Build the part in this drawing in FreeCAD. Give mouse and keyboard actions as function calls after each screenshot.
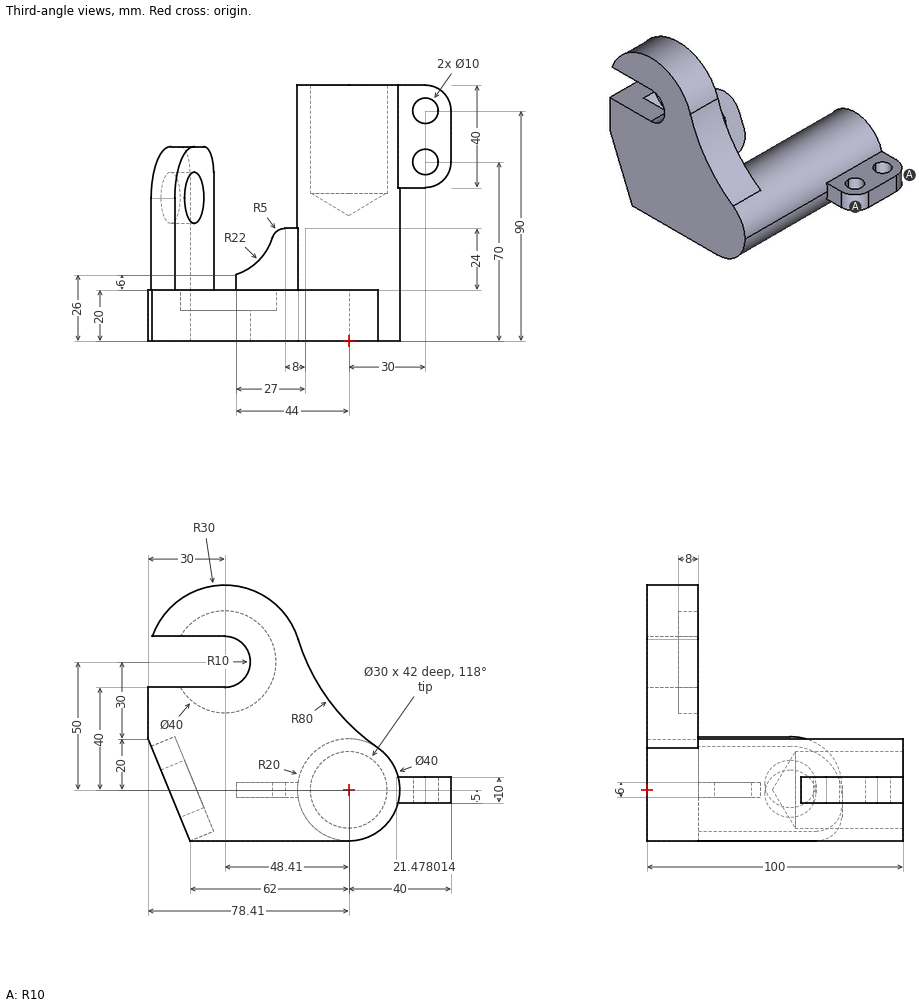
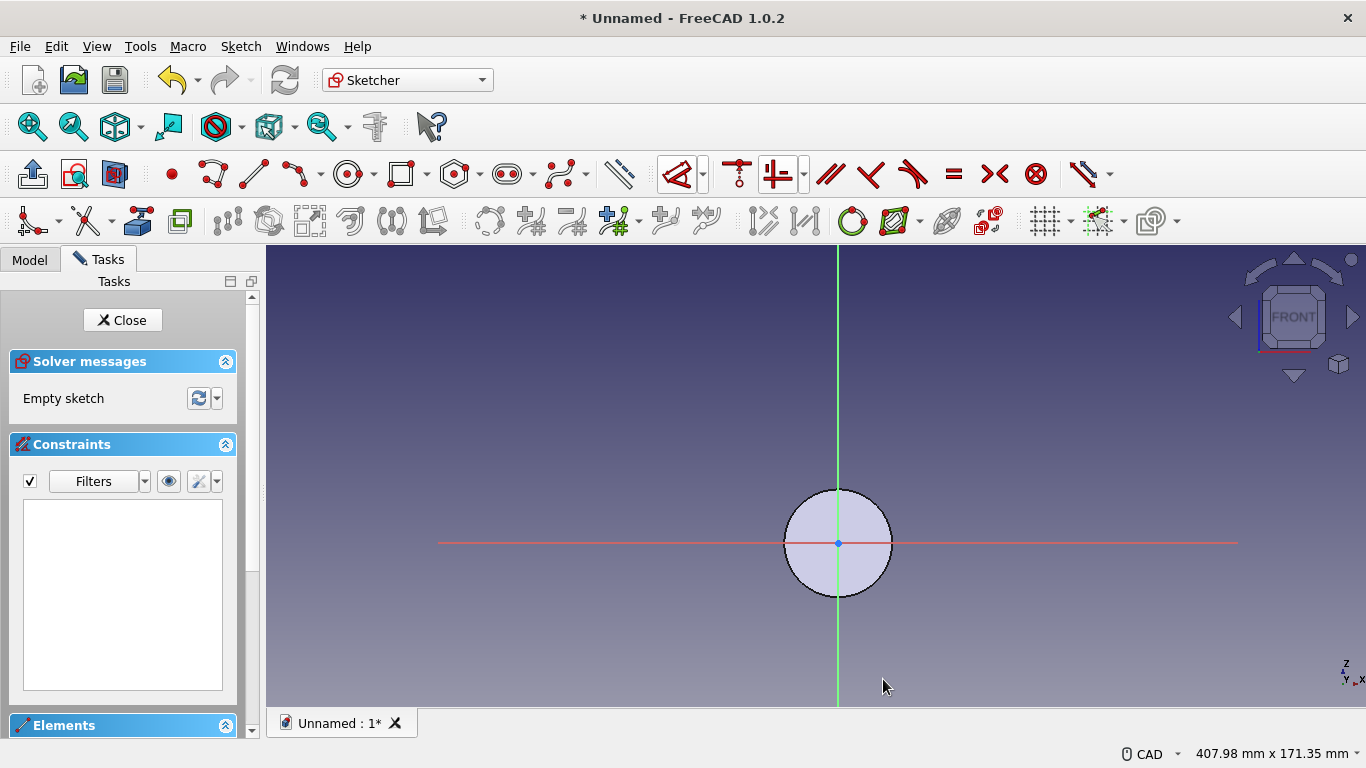
key(g)
key(m)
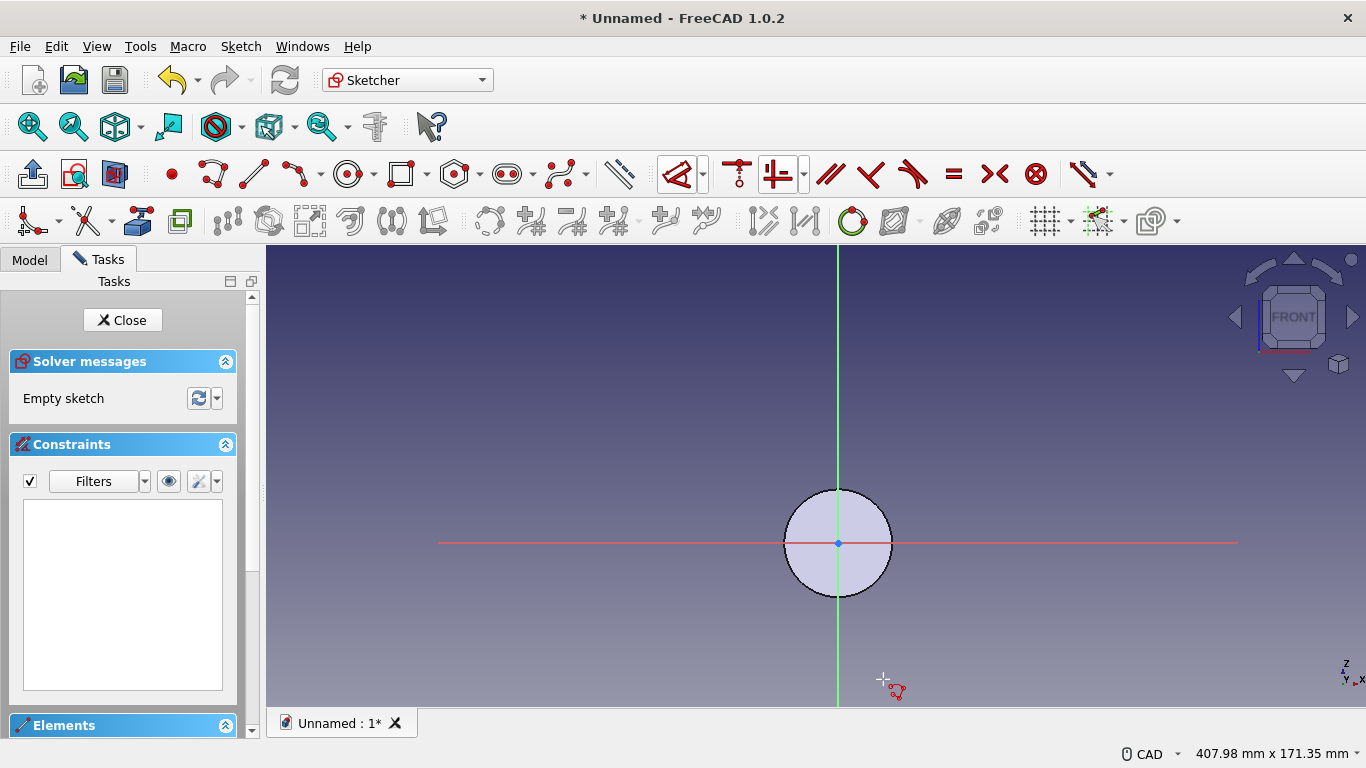
click(838, 597)
click(671, 597)
click(627, 489)
click(627, 408)
right_click(627, 408)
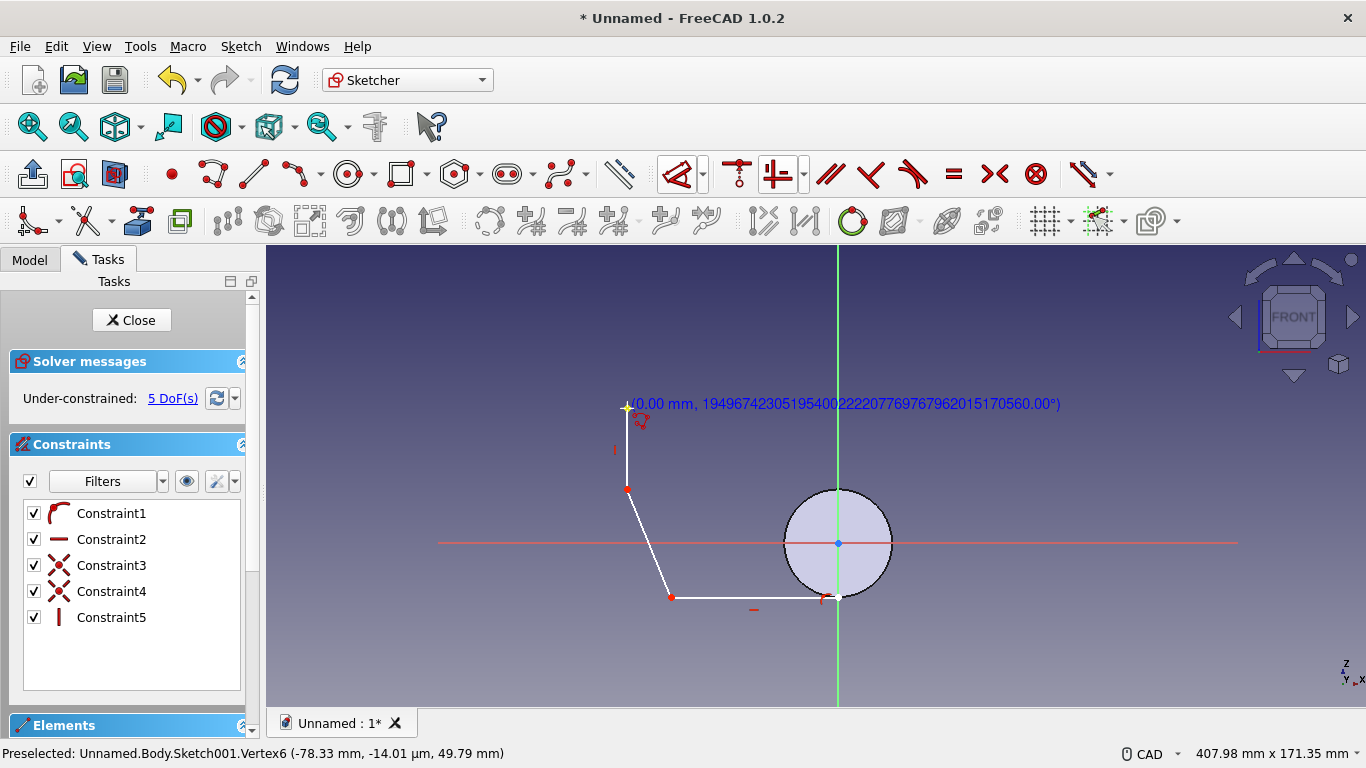
key(g)
key(3)
key(a)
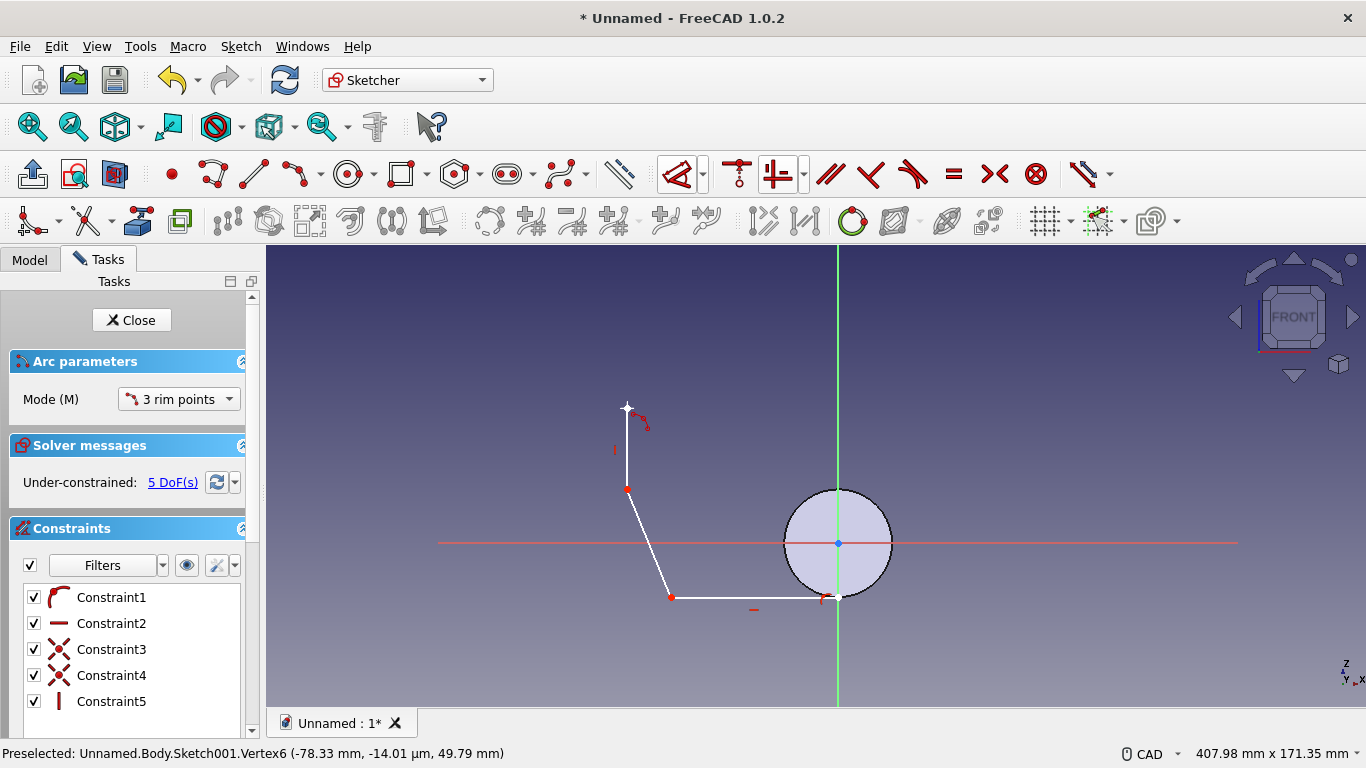
click(627, 409)
click(785, 385)
click(696, 328)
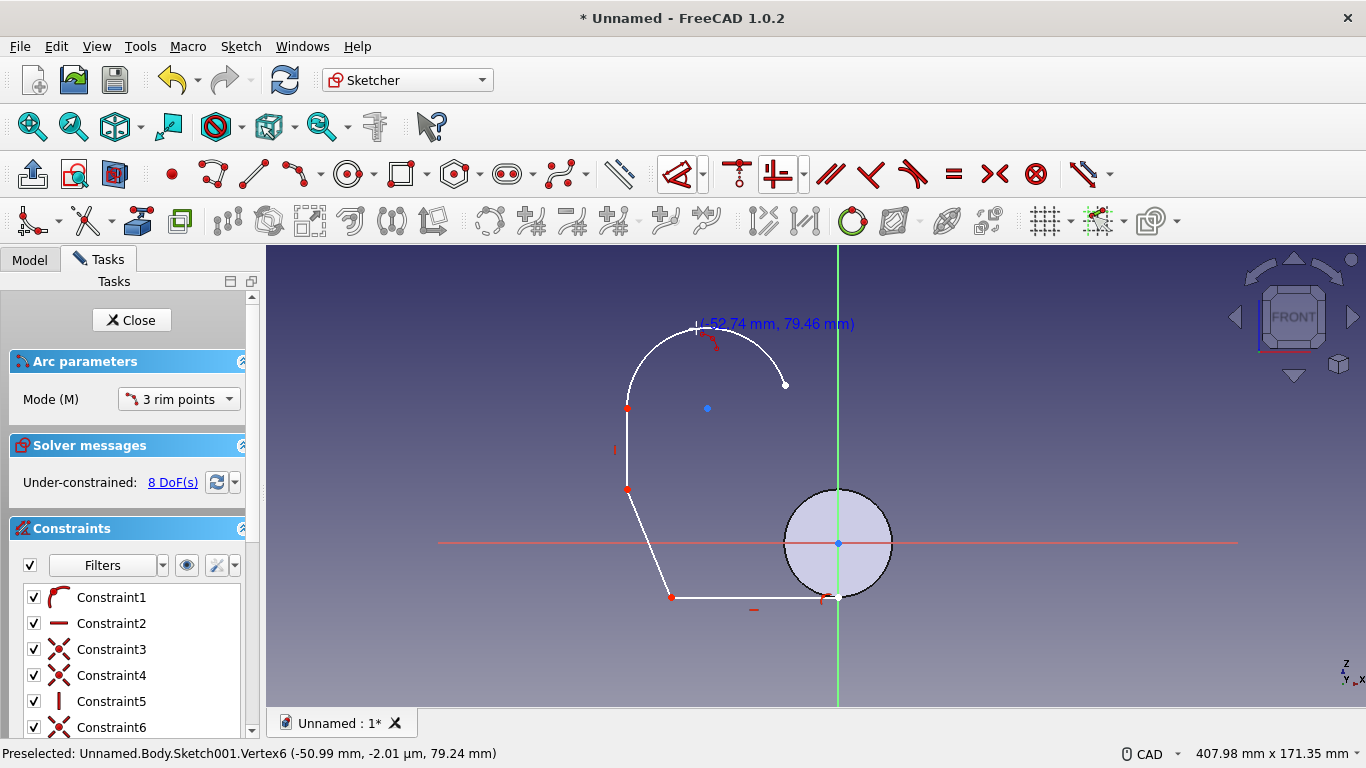
click(785, 386)
click(869, 499)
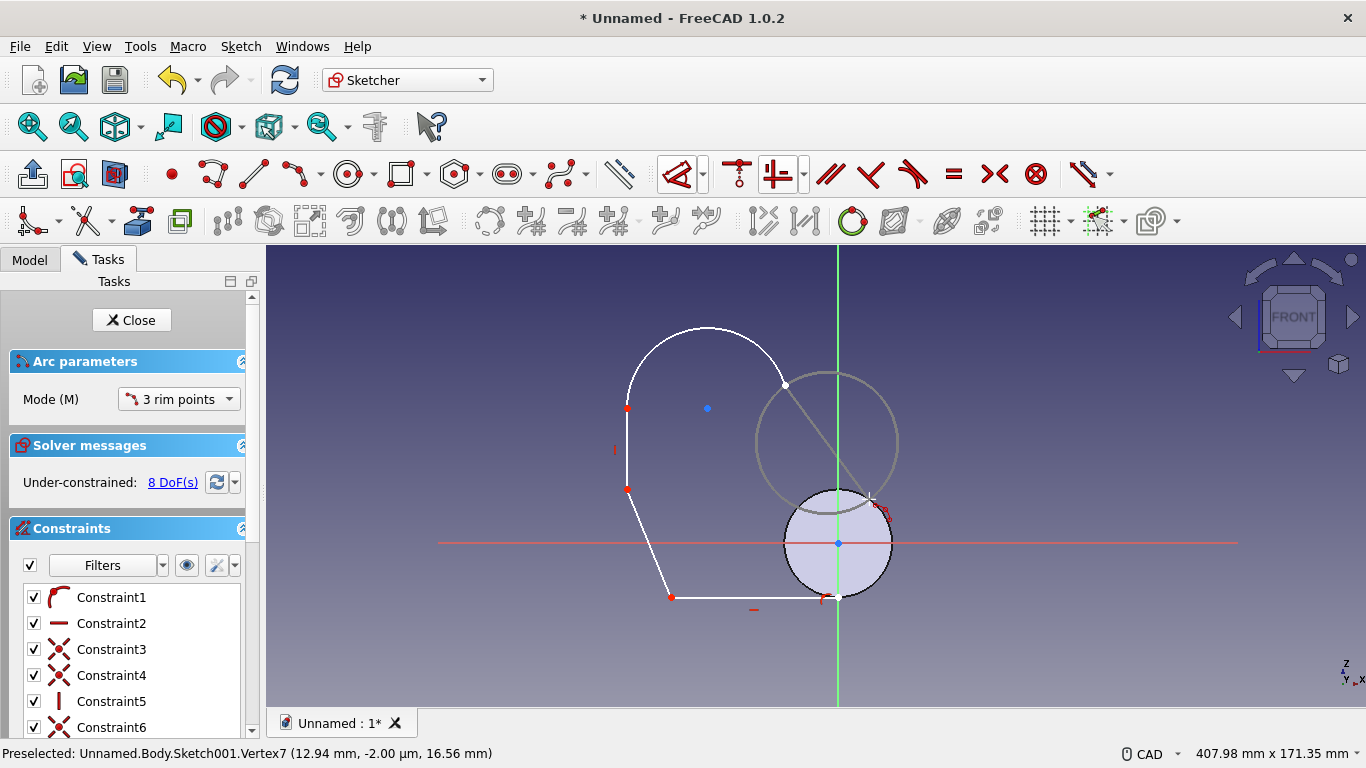
scroll(817, 449, up, 2)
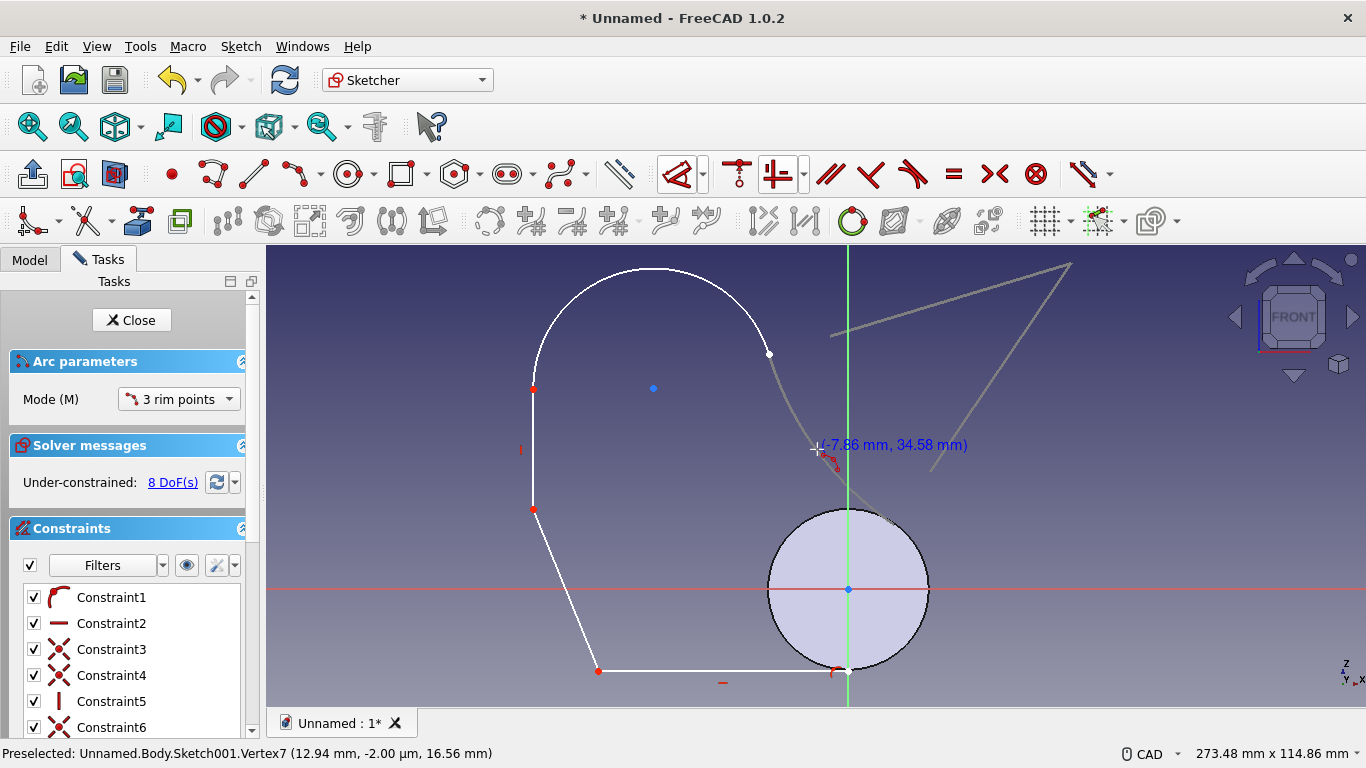
click(817, 448)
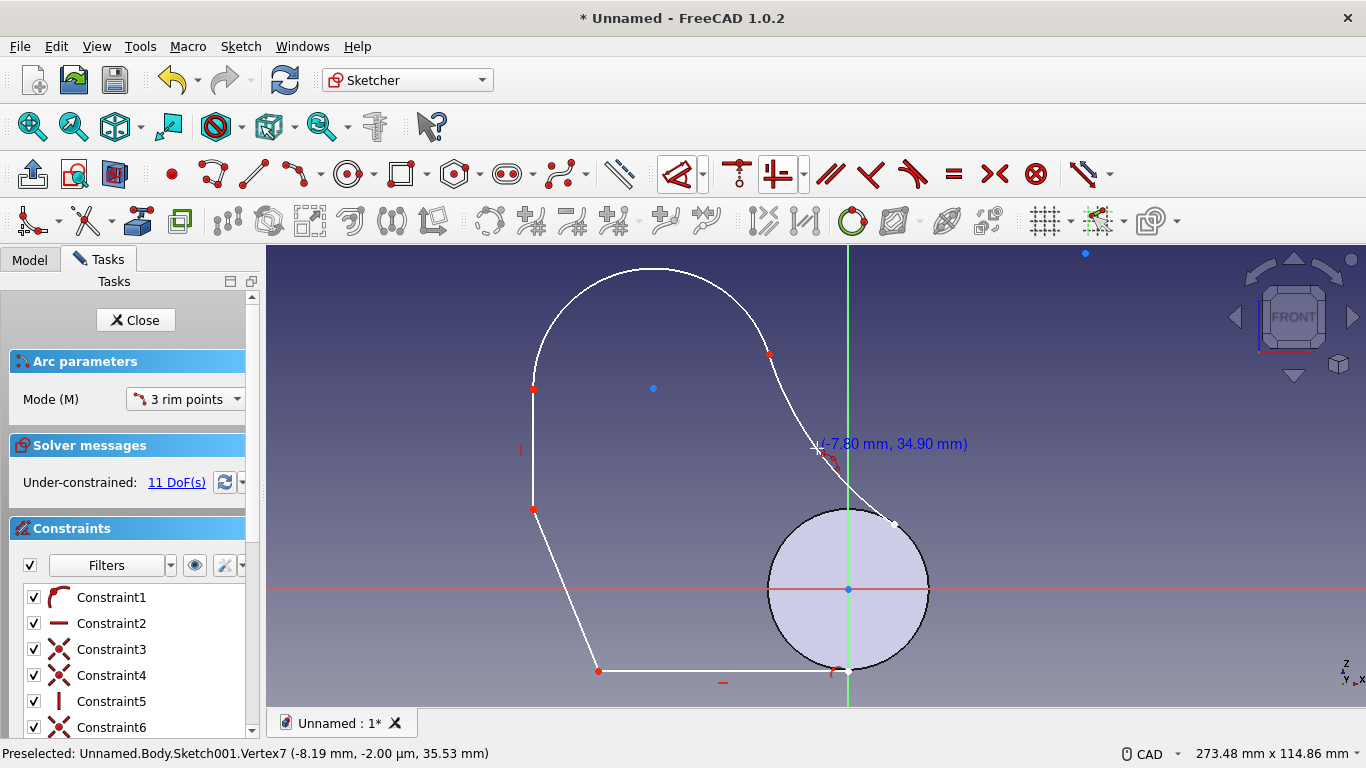
click(894, 525)
click(848, 671)
click(772, 565)
key(Escape)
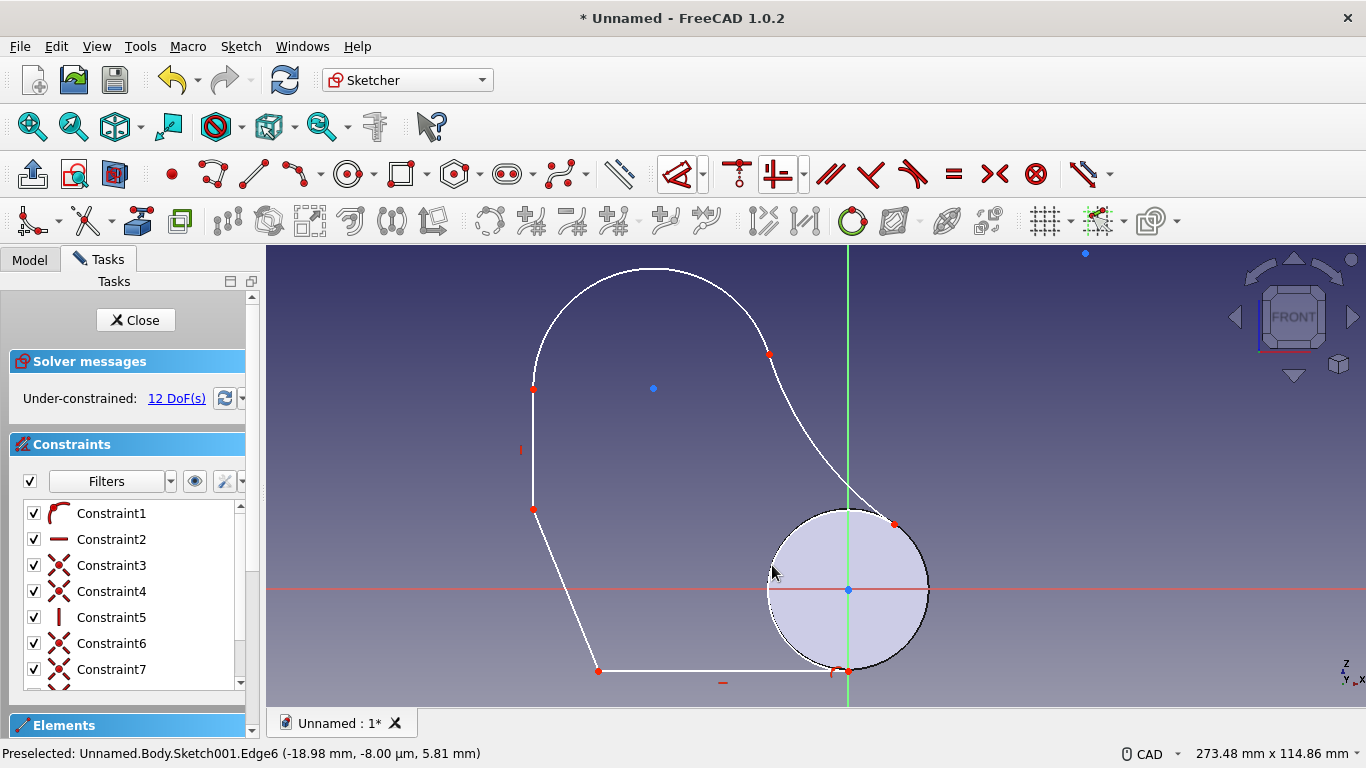
click(774, 671)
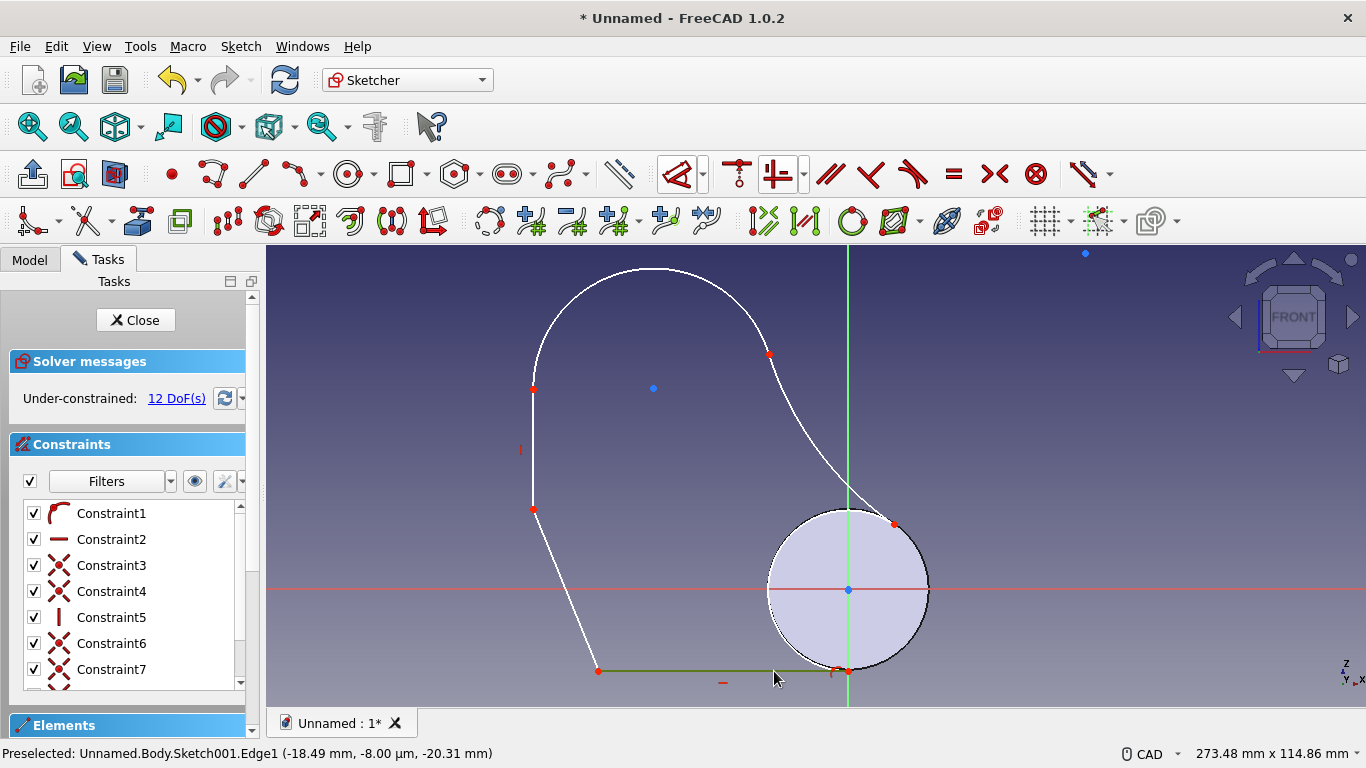
click(809, 521)